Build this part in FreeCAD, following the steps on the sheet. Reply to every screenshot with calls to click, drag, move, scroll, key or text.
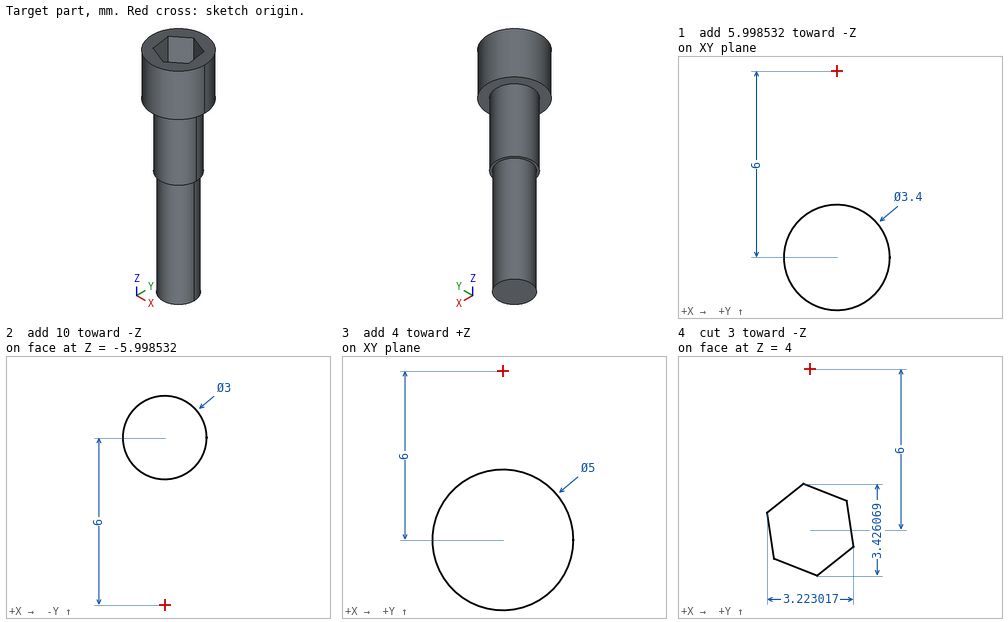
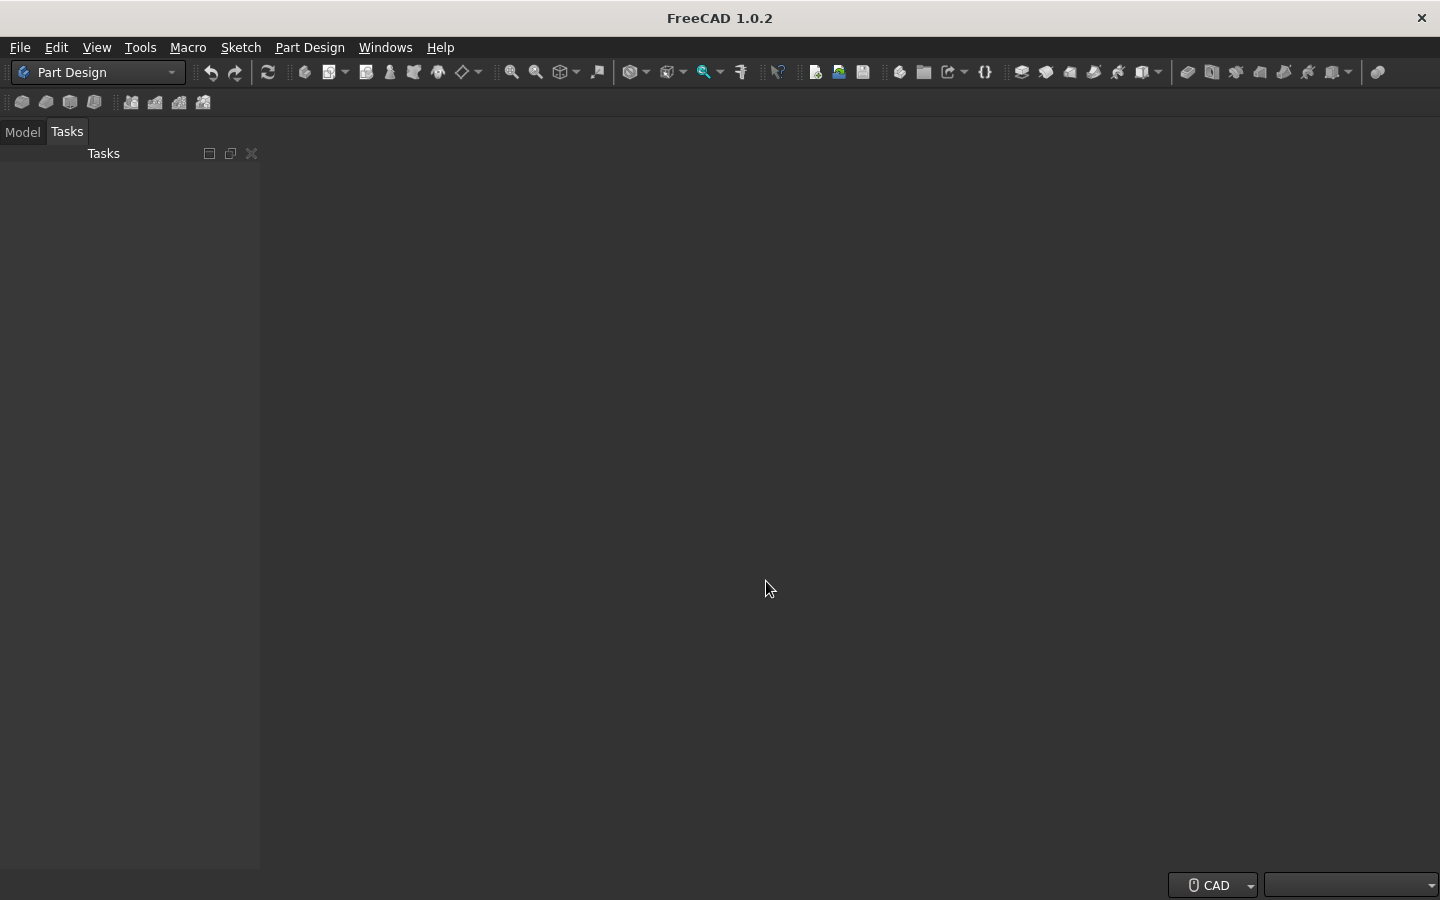
key(ctrl+n)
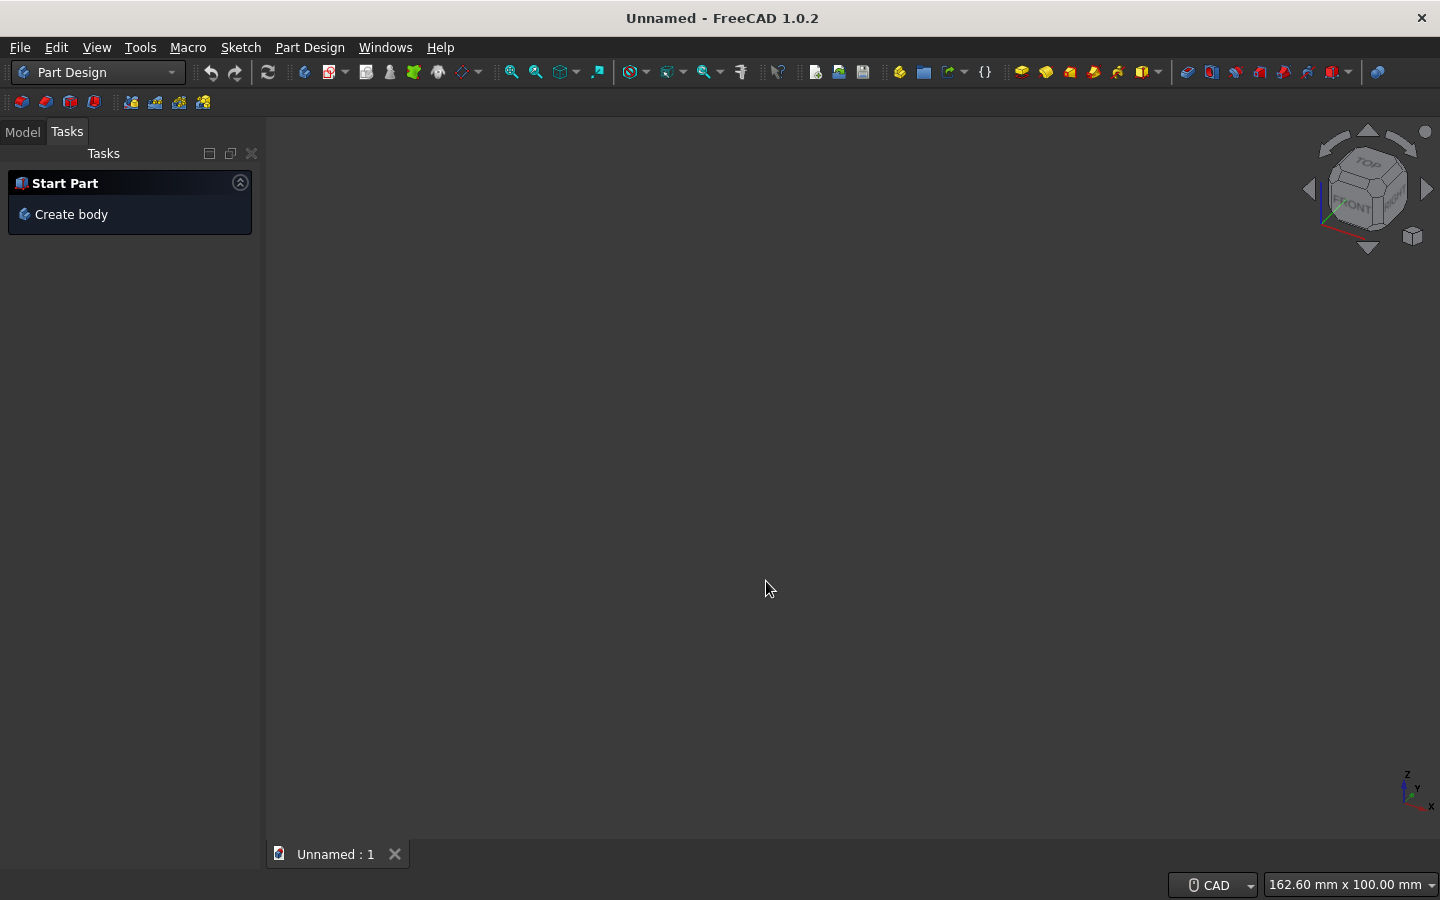
click(330, 72)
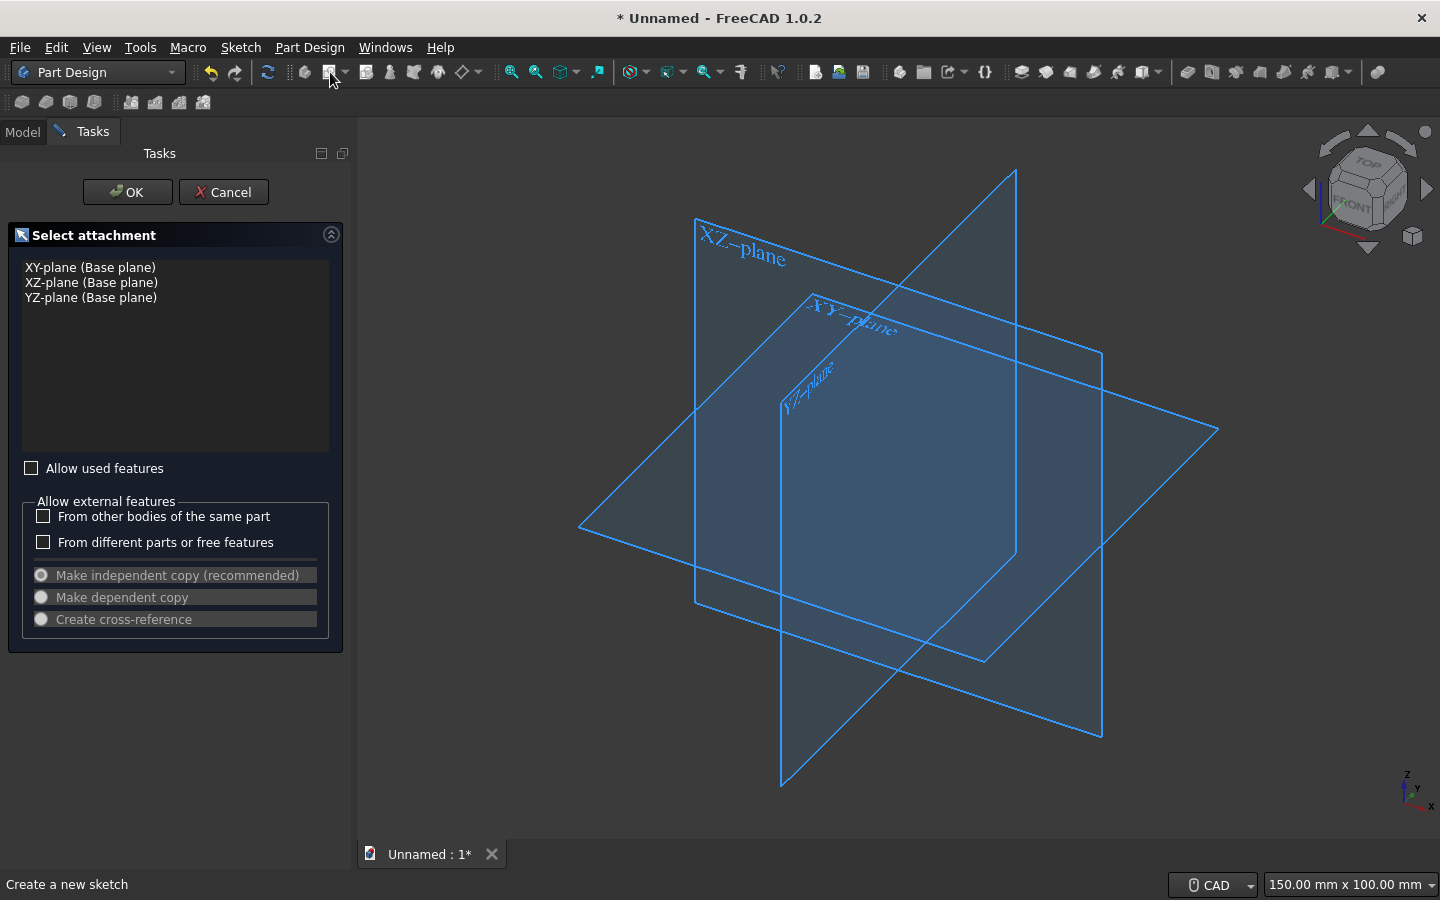
click(82, 268)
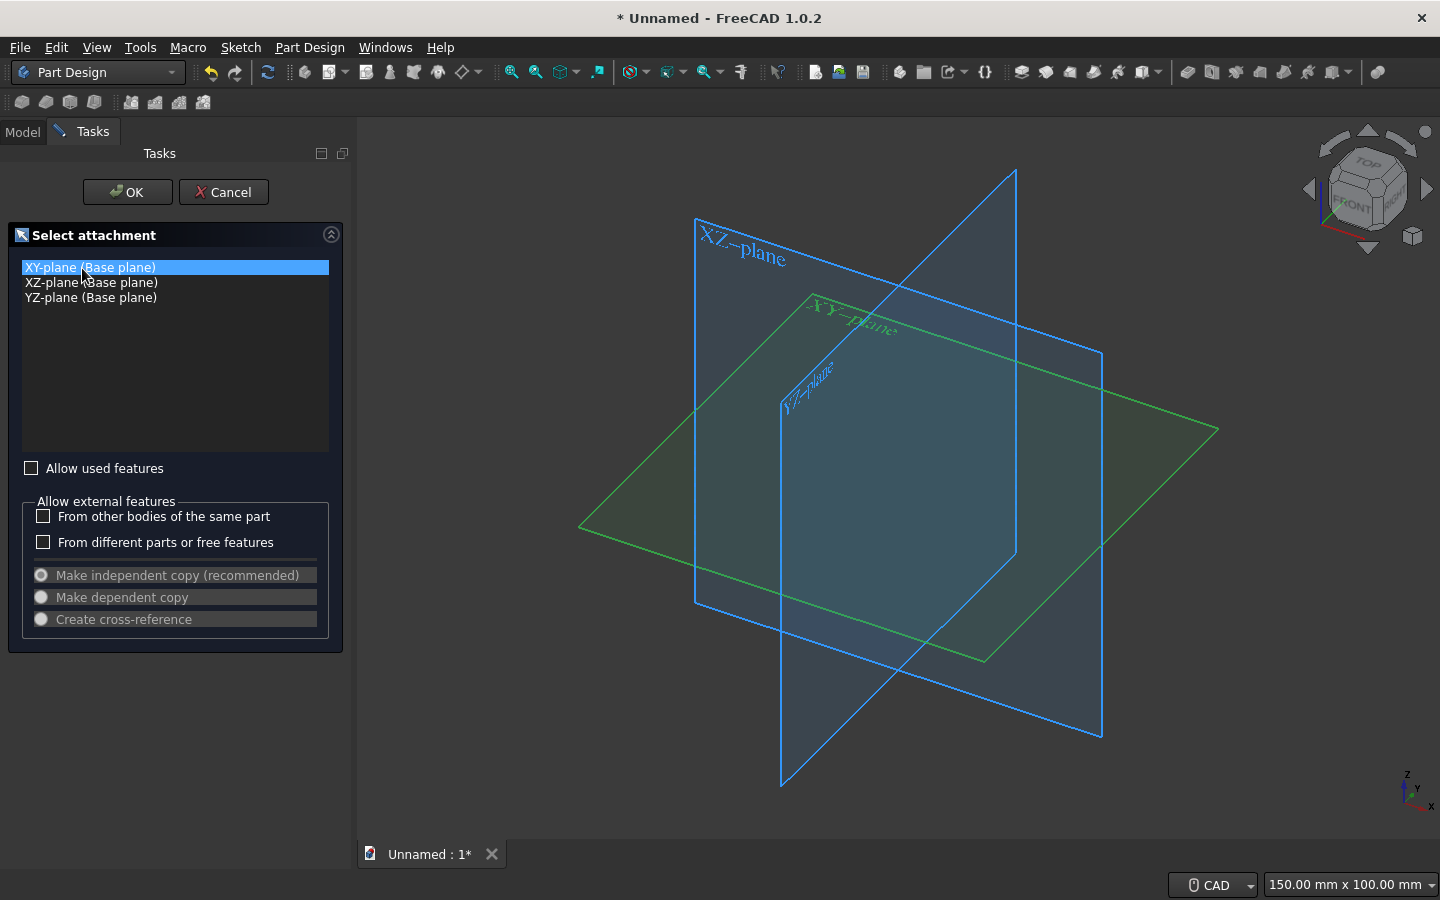
click(128, 192)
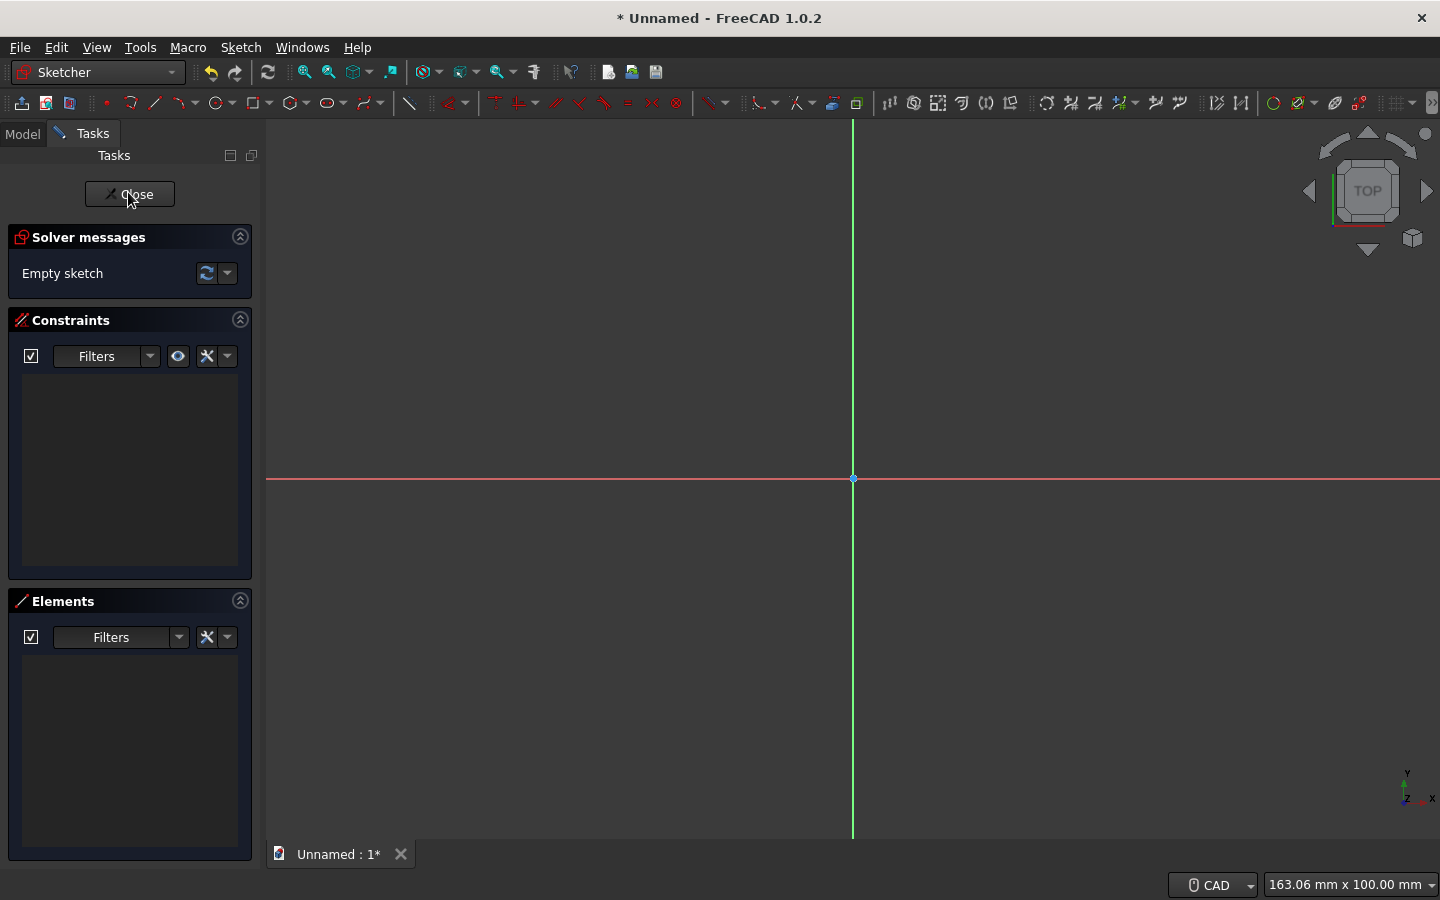
scroll(862, 510, up, 11)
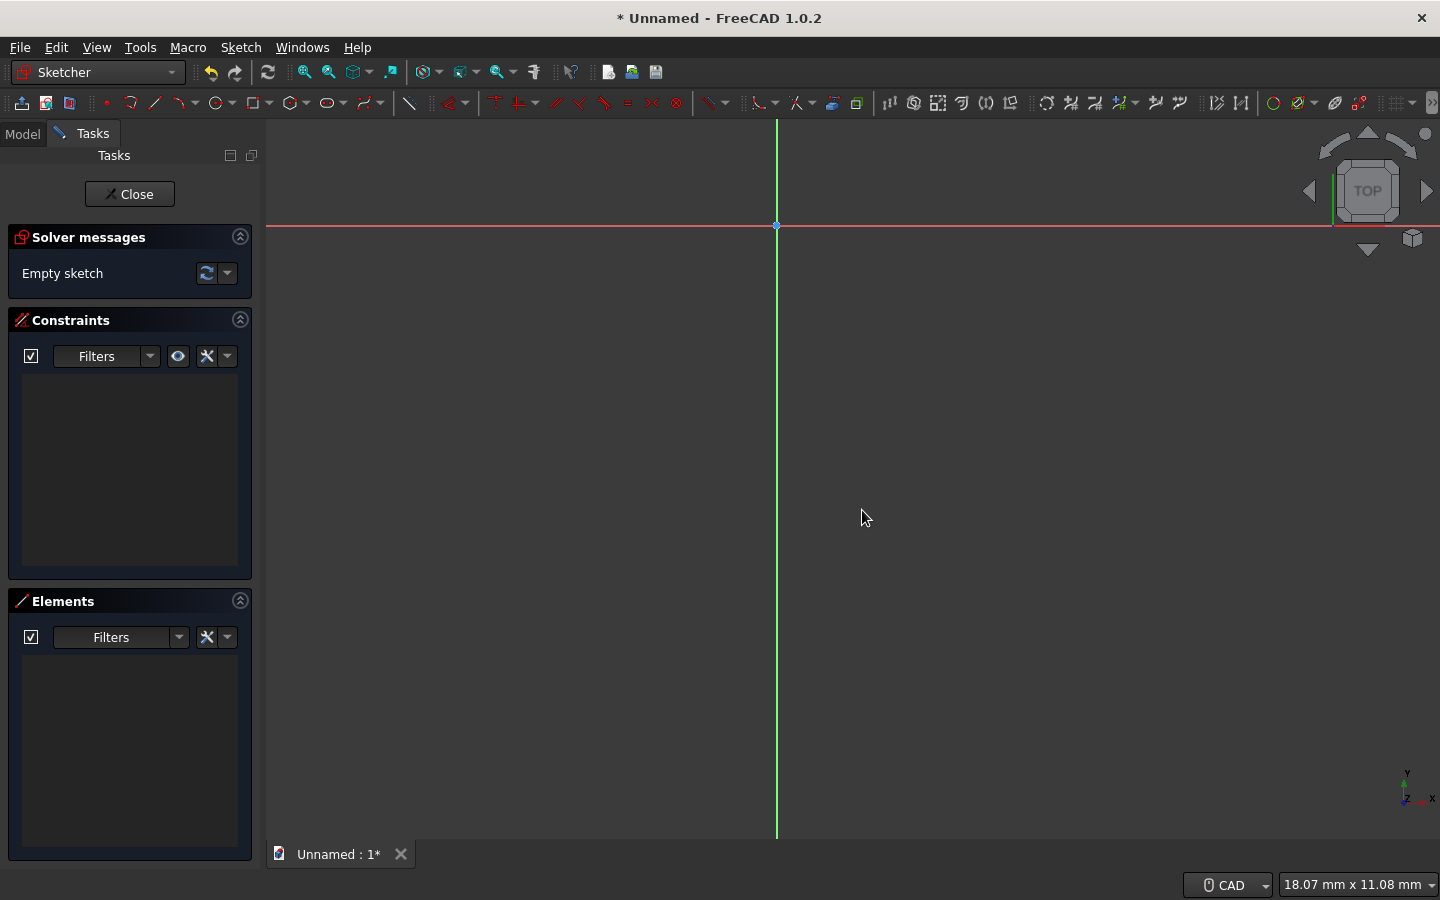
key(g)
key(c)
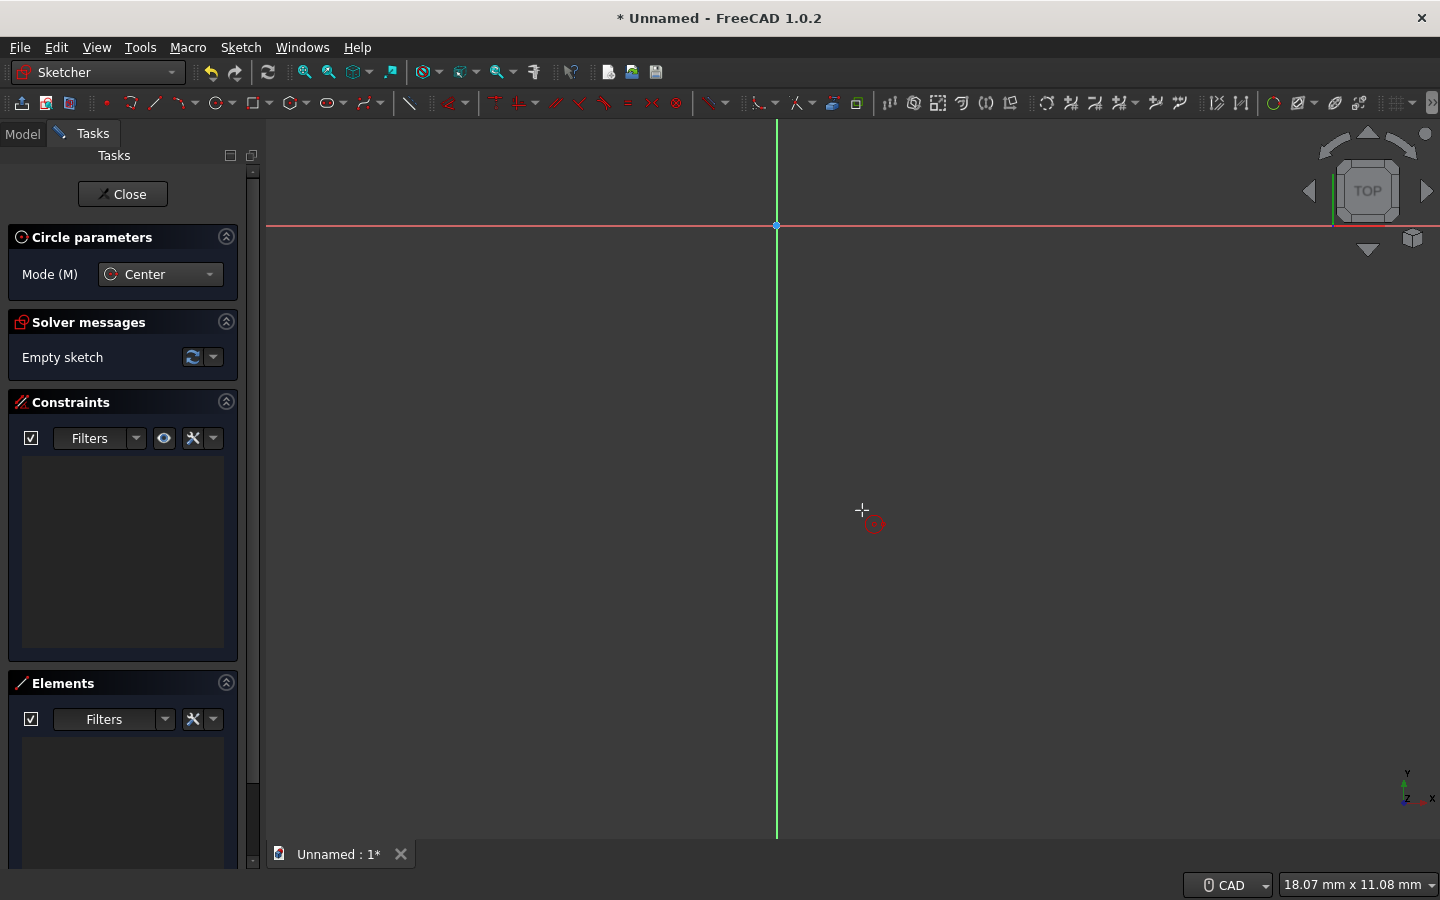
click(777, 616)
click(855, 538)
key(Escape)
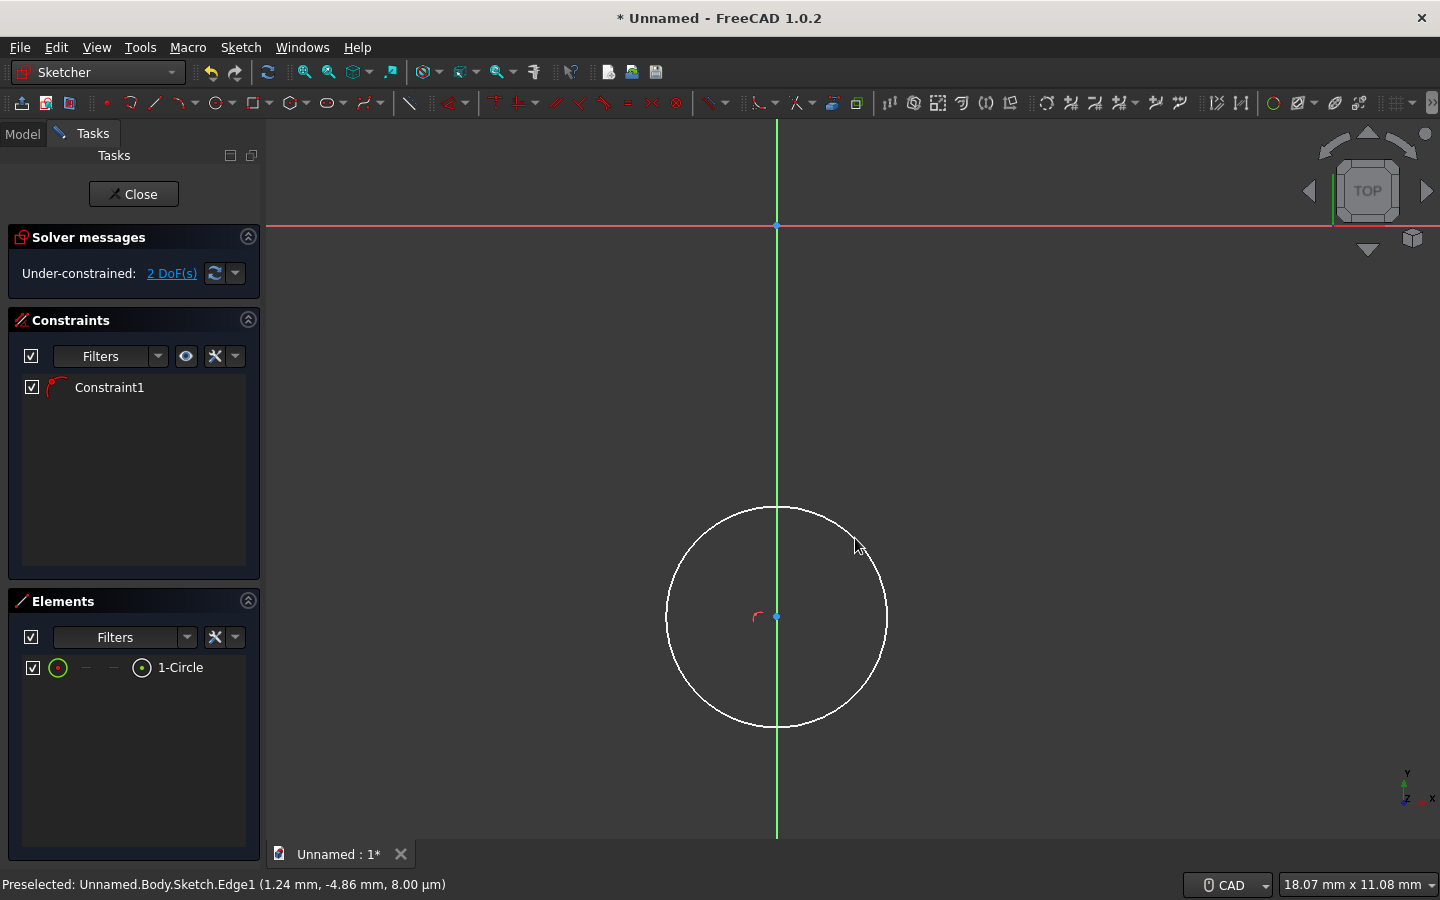
key(d)